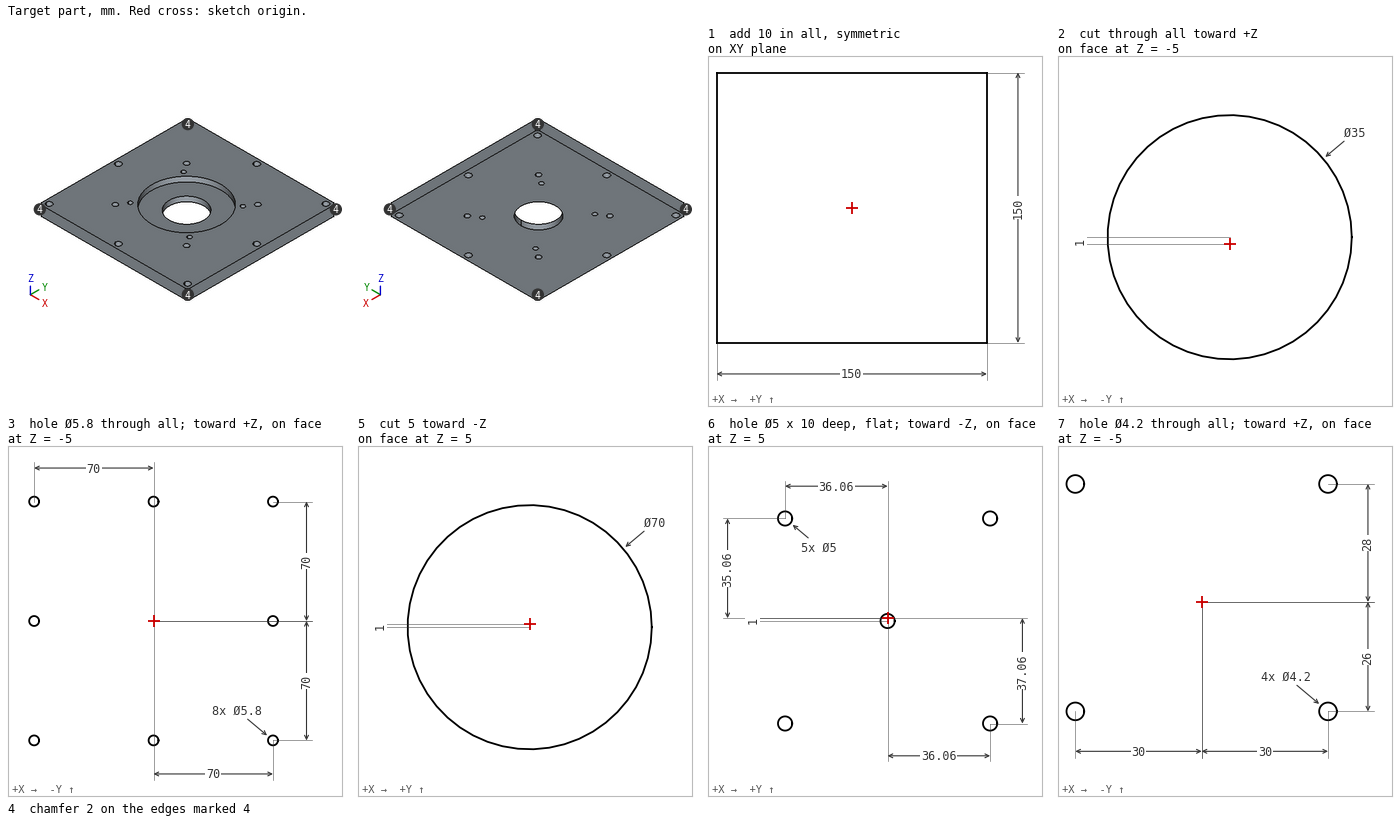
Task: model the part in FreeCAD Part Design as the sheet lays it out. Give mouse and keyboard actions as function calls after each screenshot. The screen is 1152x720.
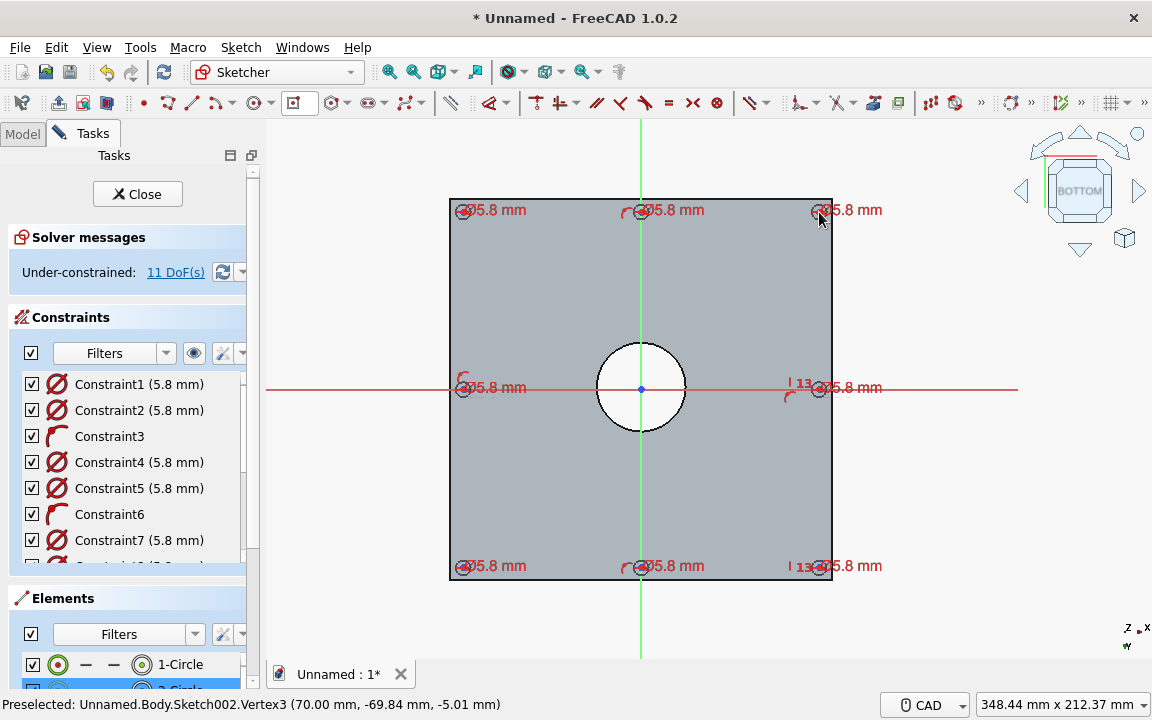
key(v)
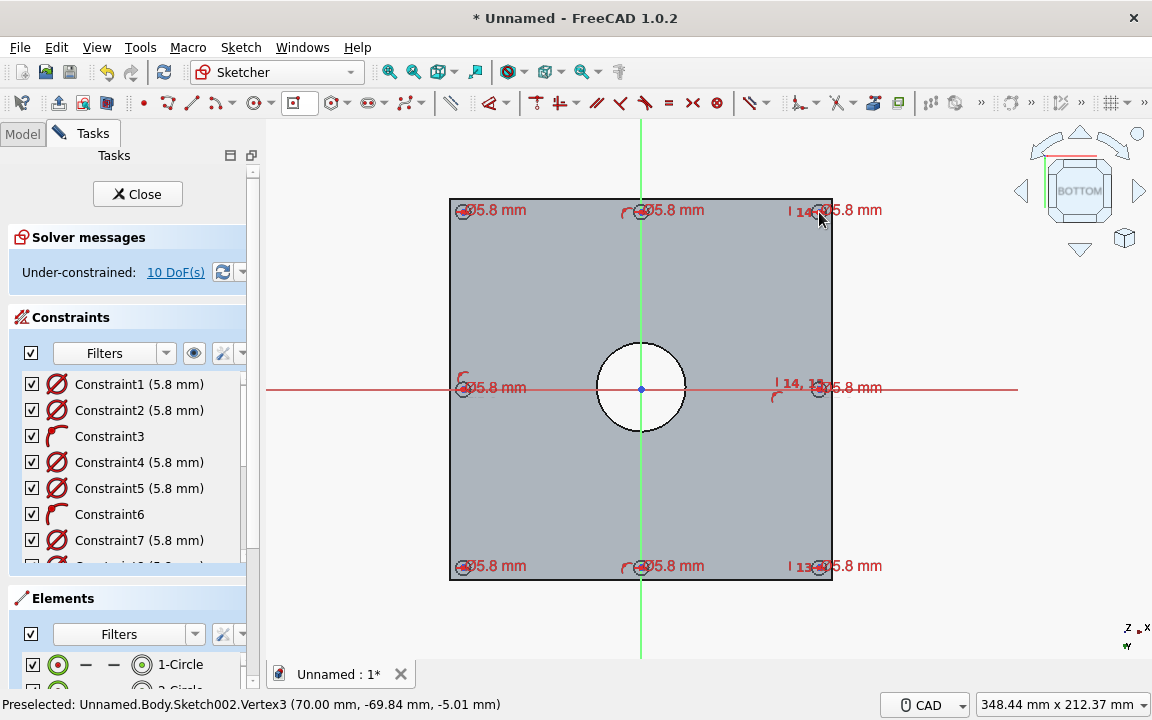
click(819, 212)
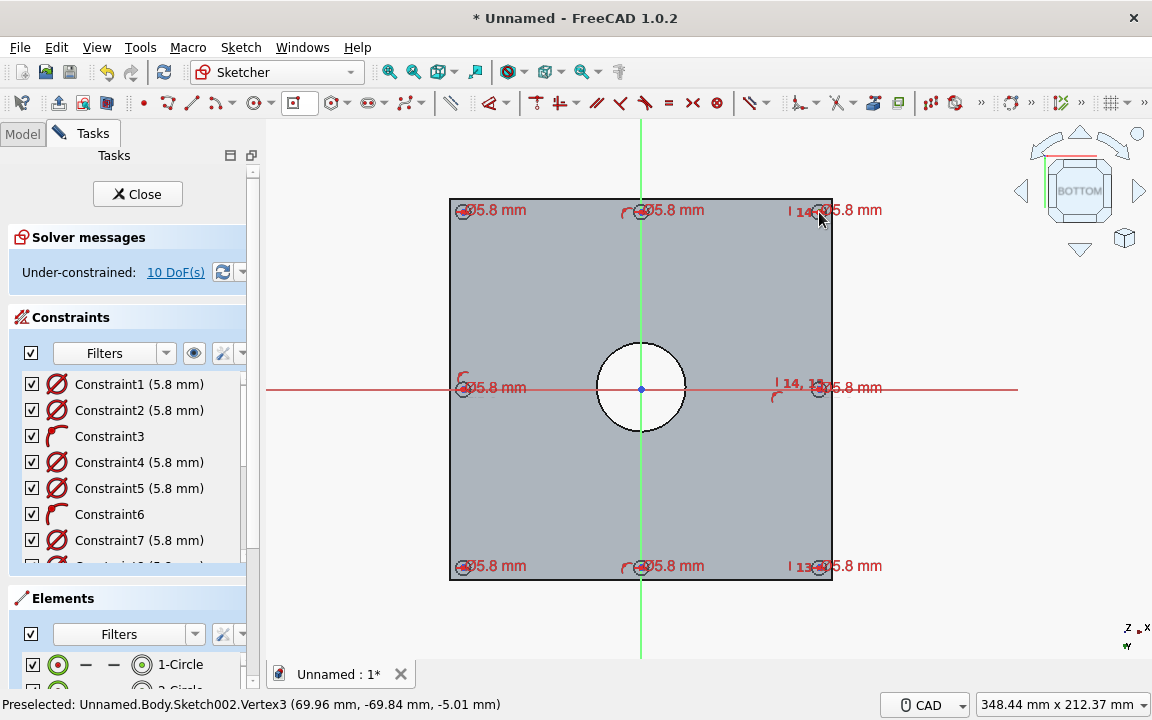
click(641, 212)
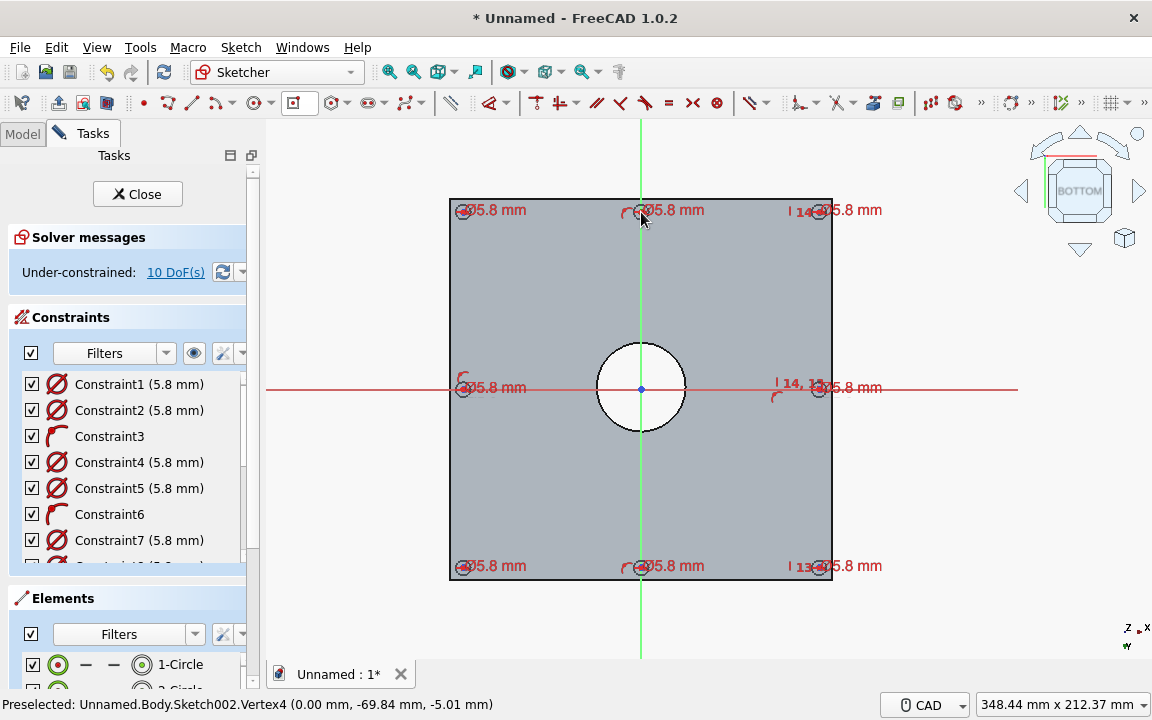
click(578, 104)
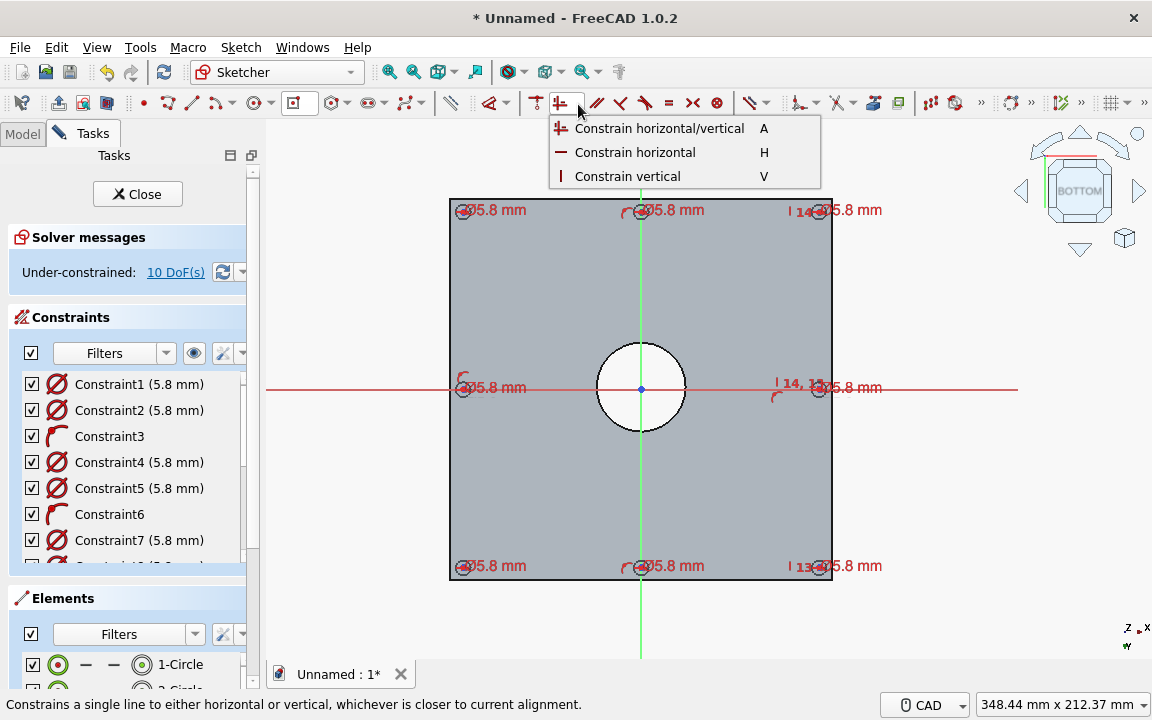
click(685, 152)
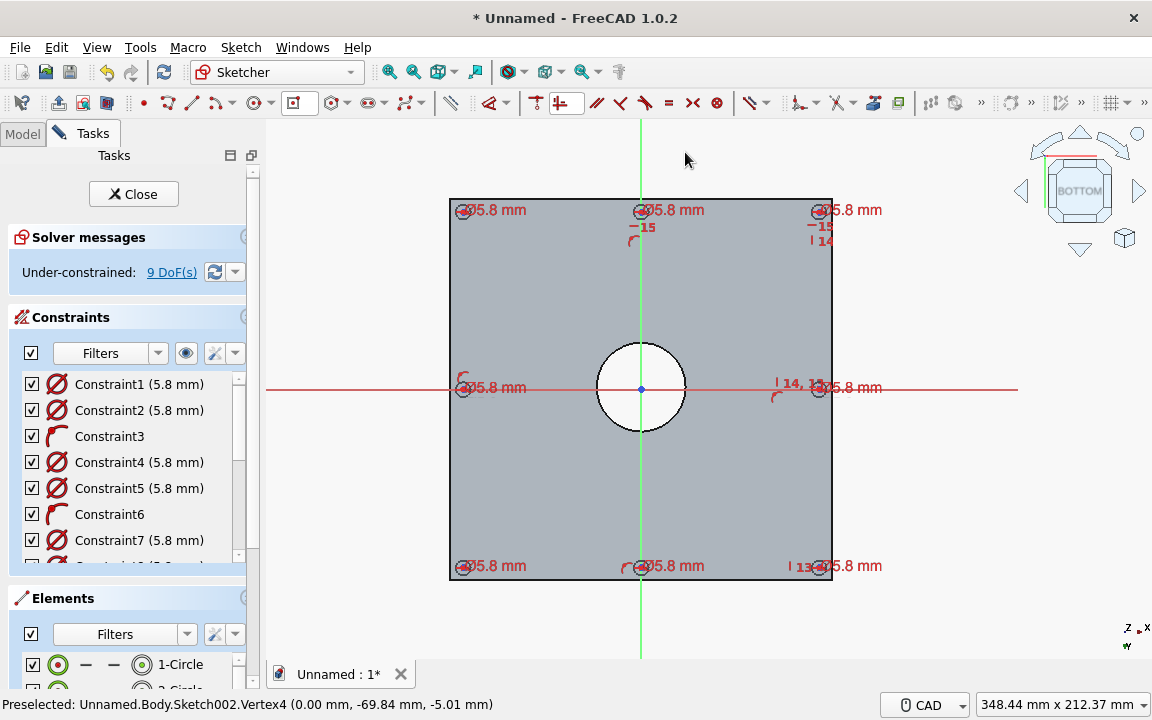
click(641, 212)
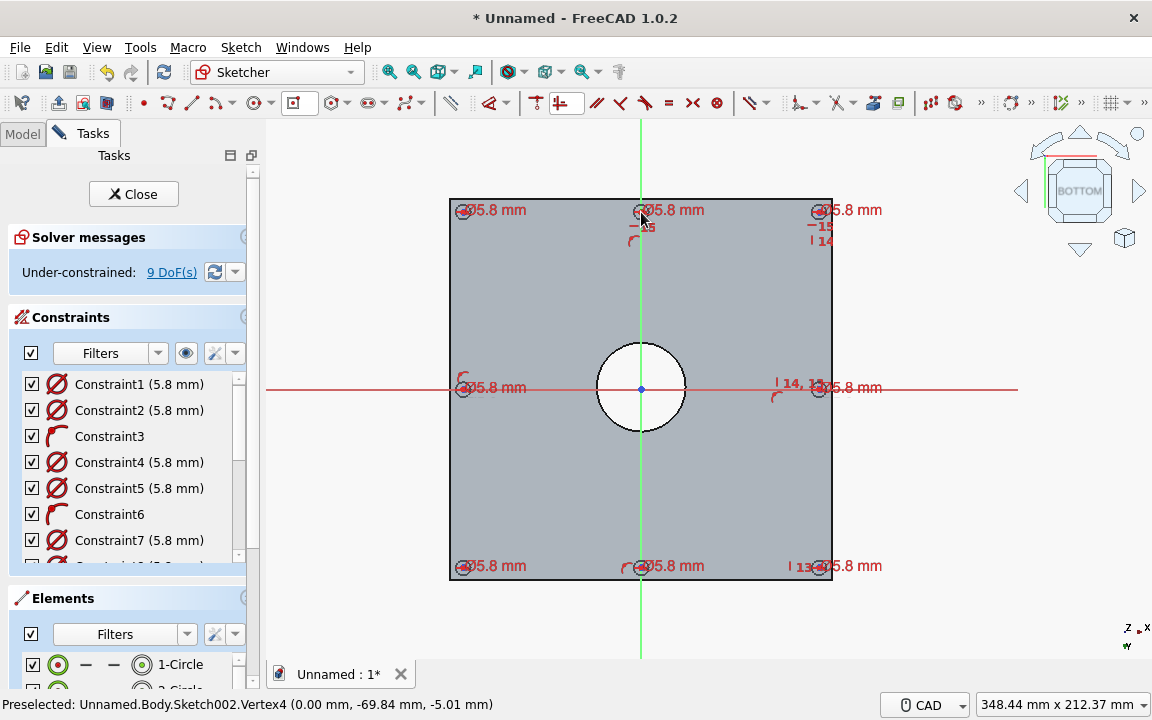
click(463, 212)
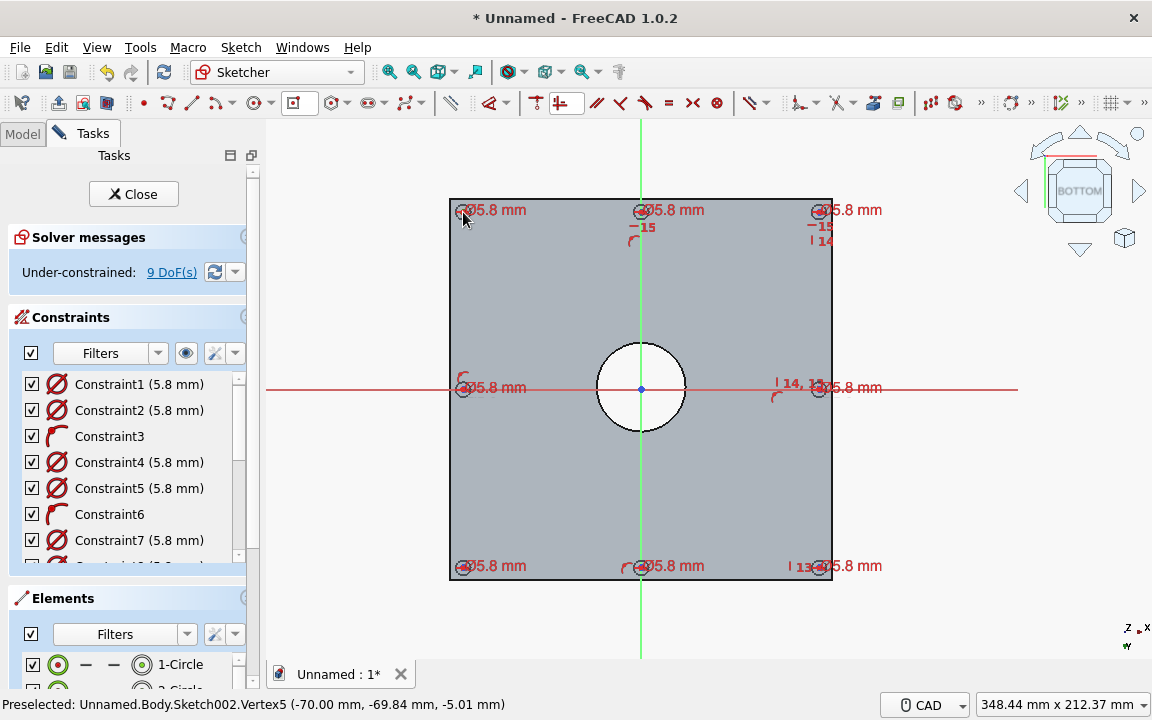
key(h)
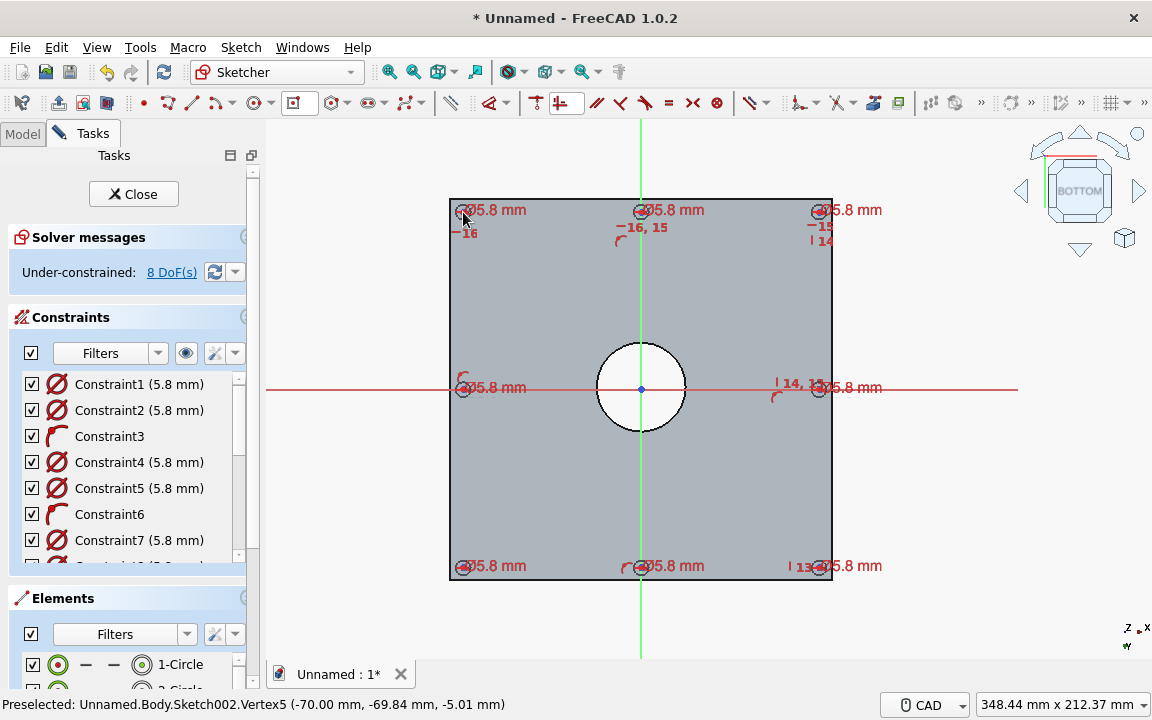
click(463, 212)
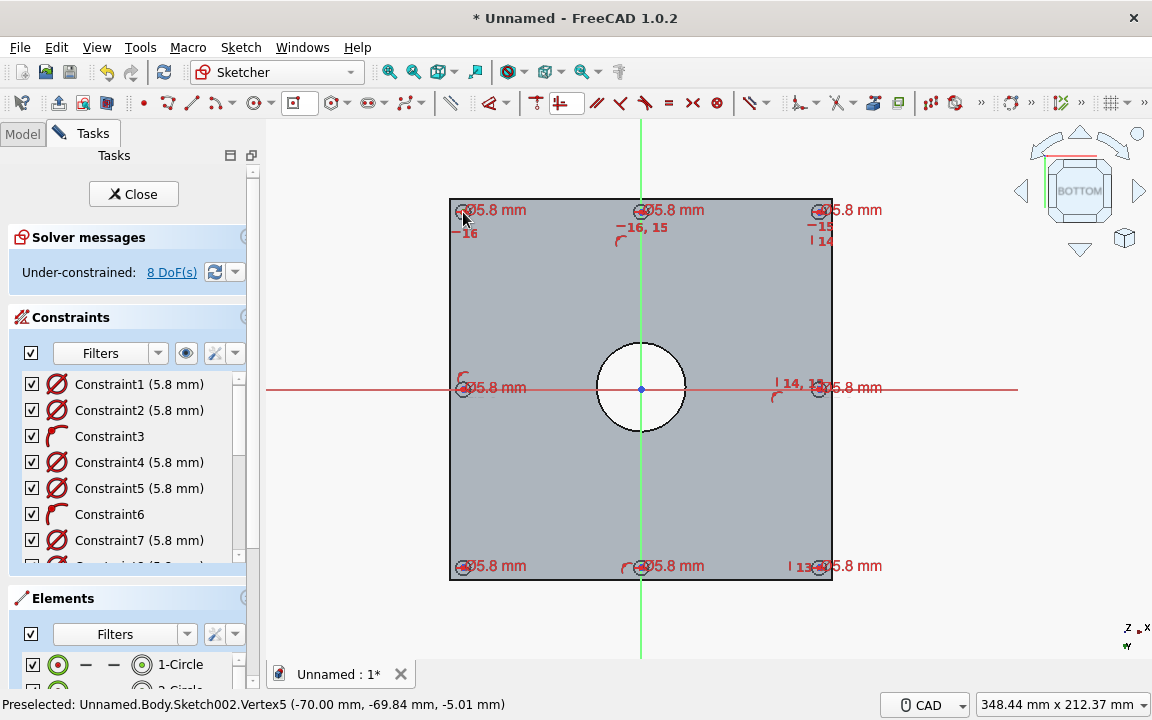
click(463, 390)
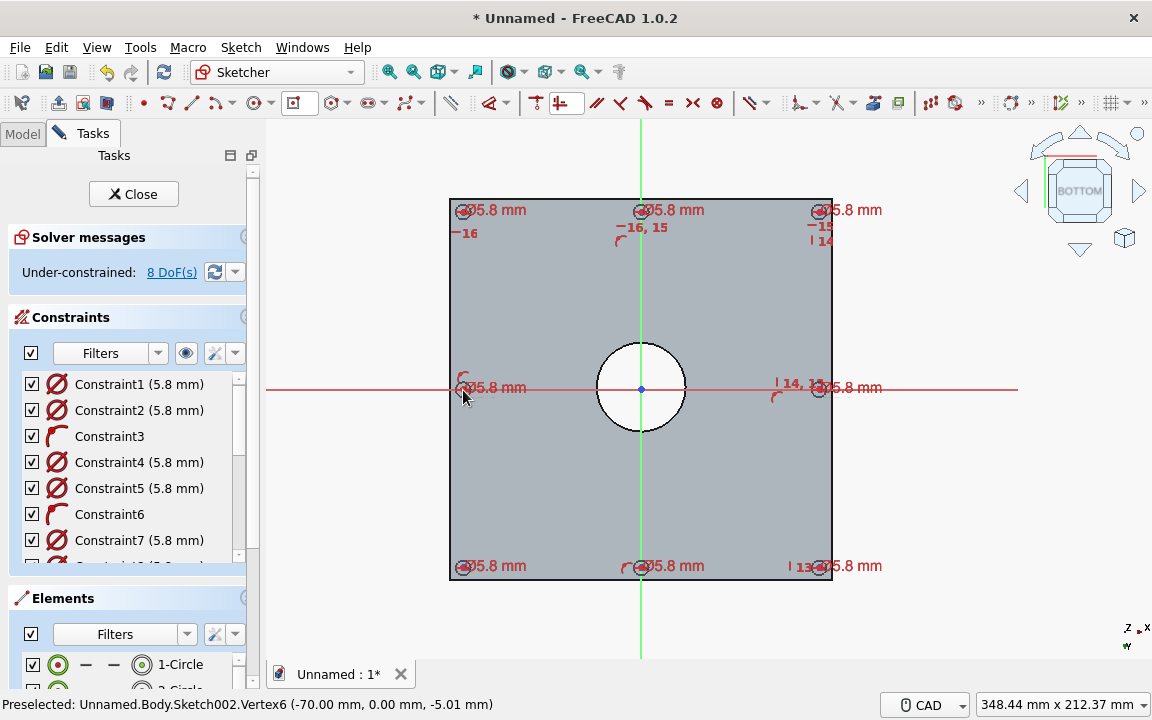
key(v)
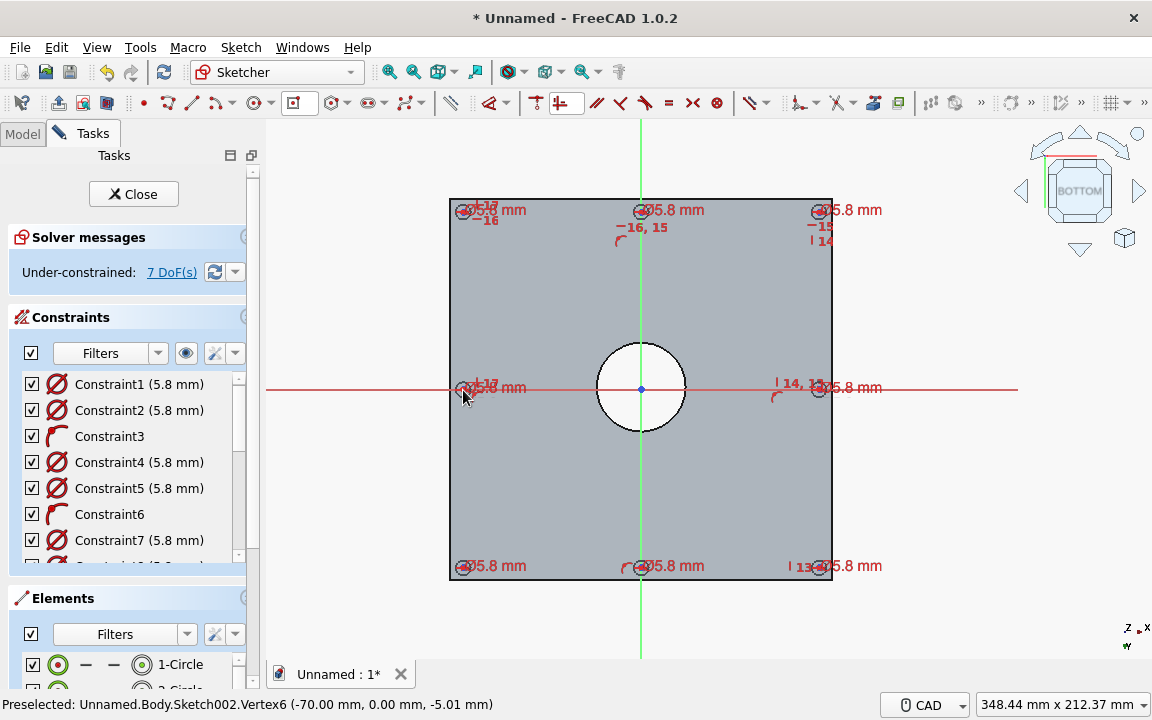
click(463, 390)